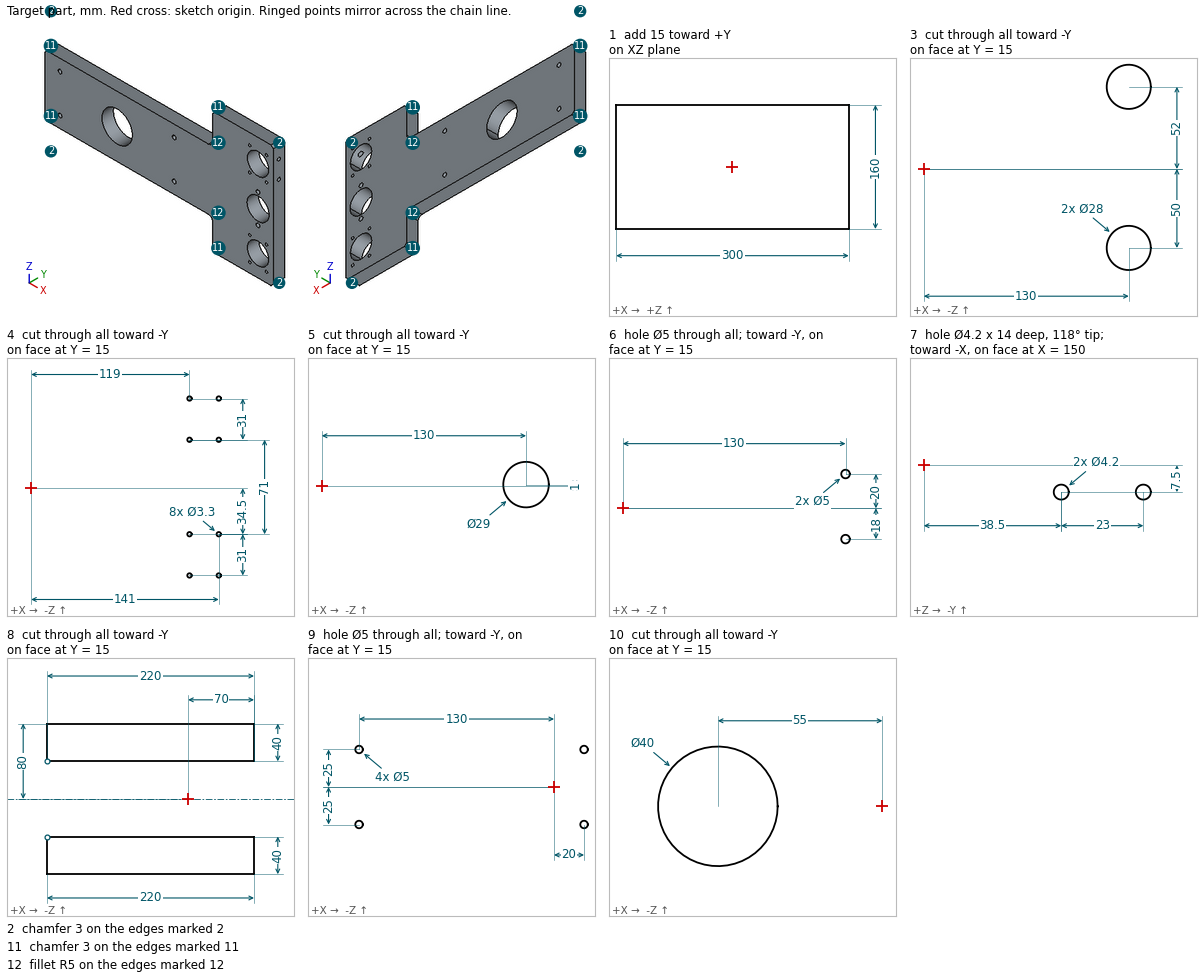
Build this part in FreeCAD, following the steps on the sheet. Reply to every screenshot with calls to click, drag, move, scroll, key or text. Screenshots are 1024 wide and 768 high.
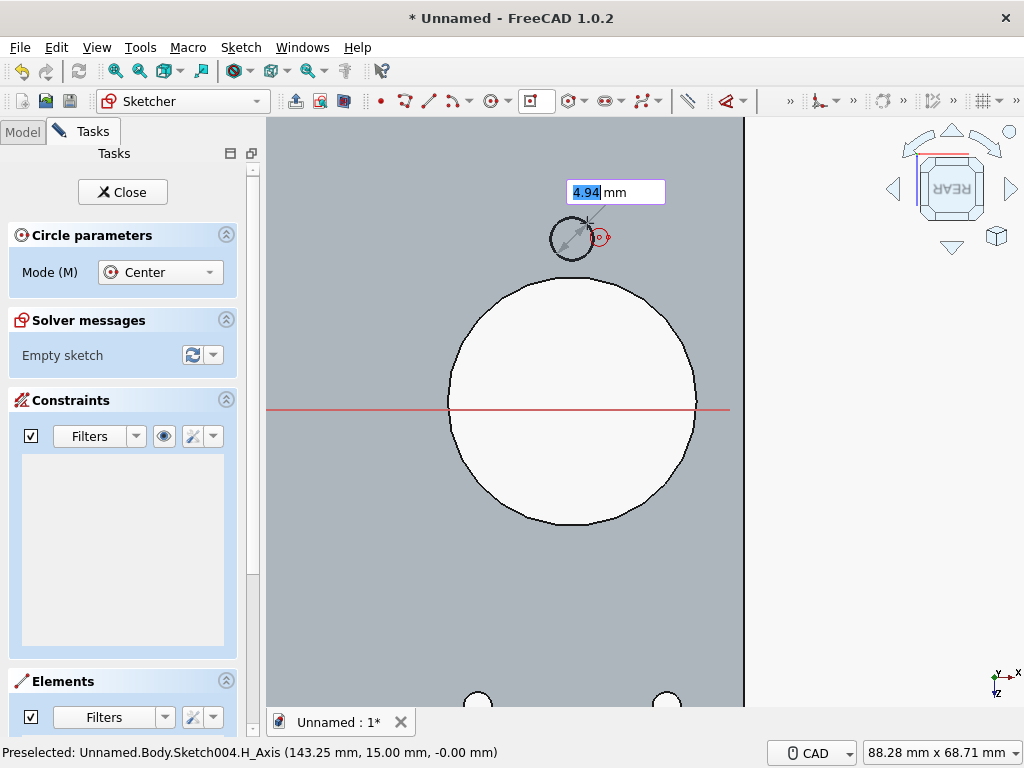
text(5)
key(Return)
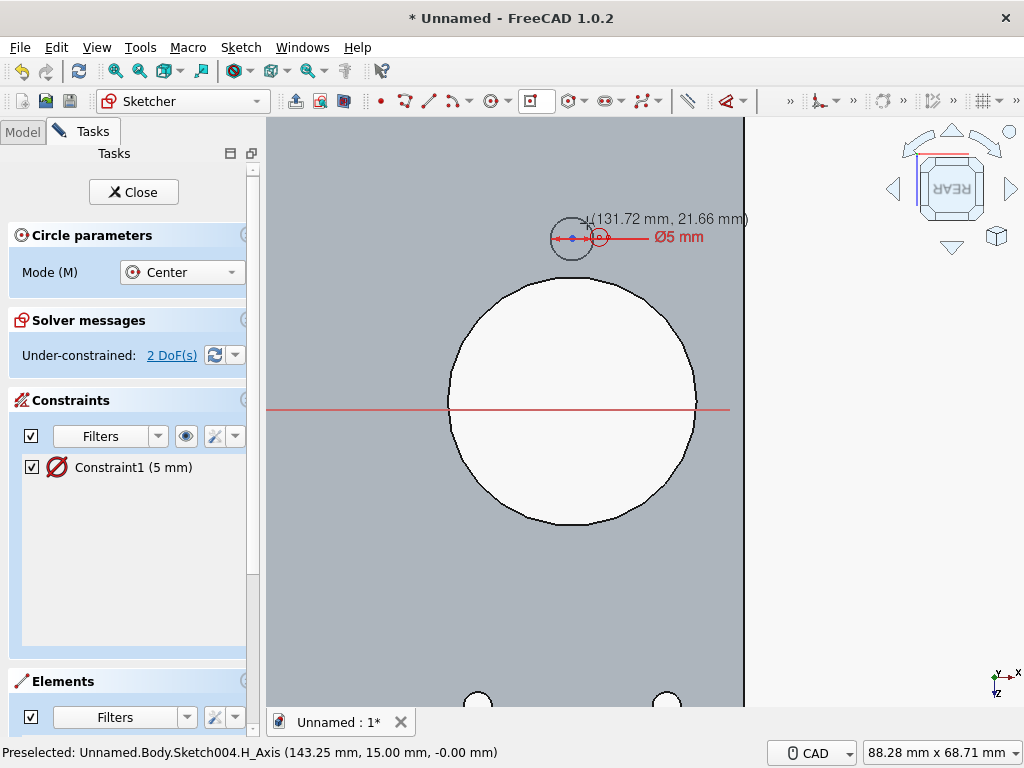
click(572, 565)
move(587, 549)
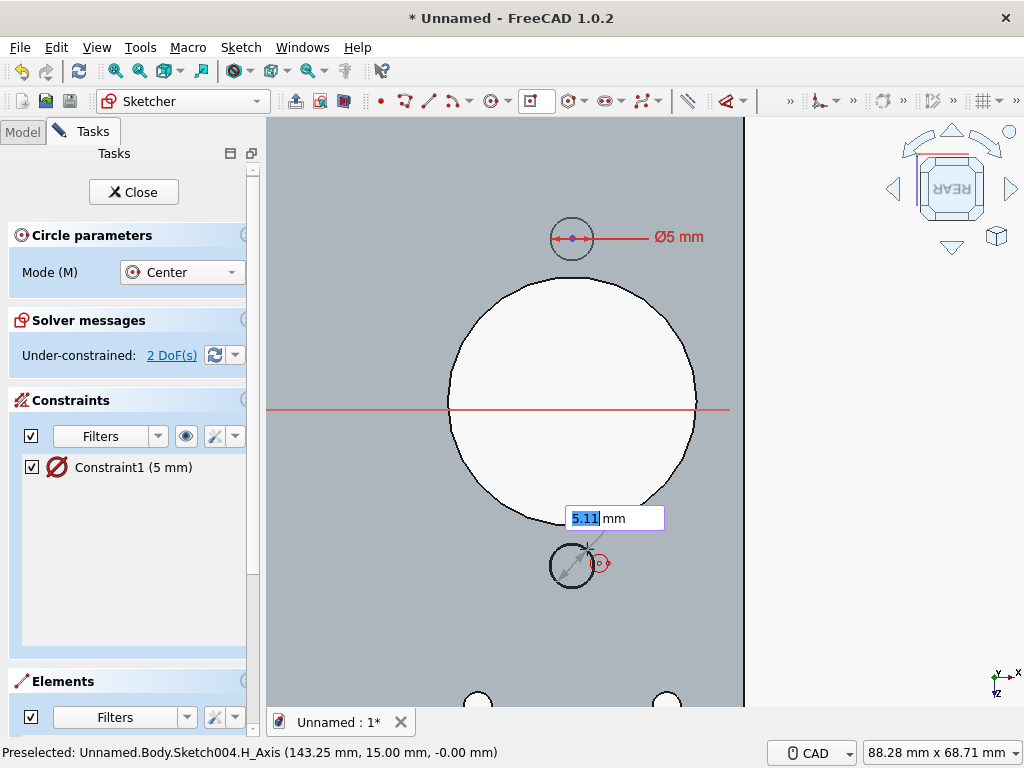
text(5)
key(Return)
key(Escape)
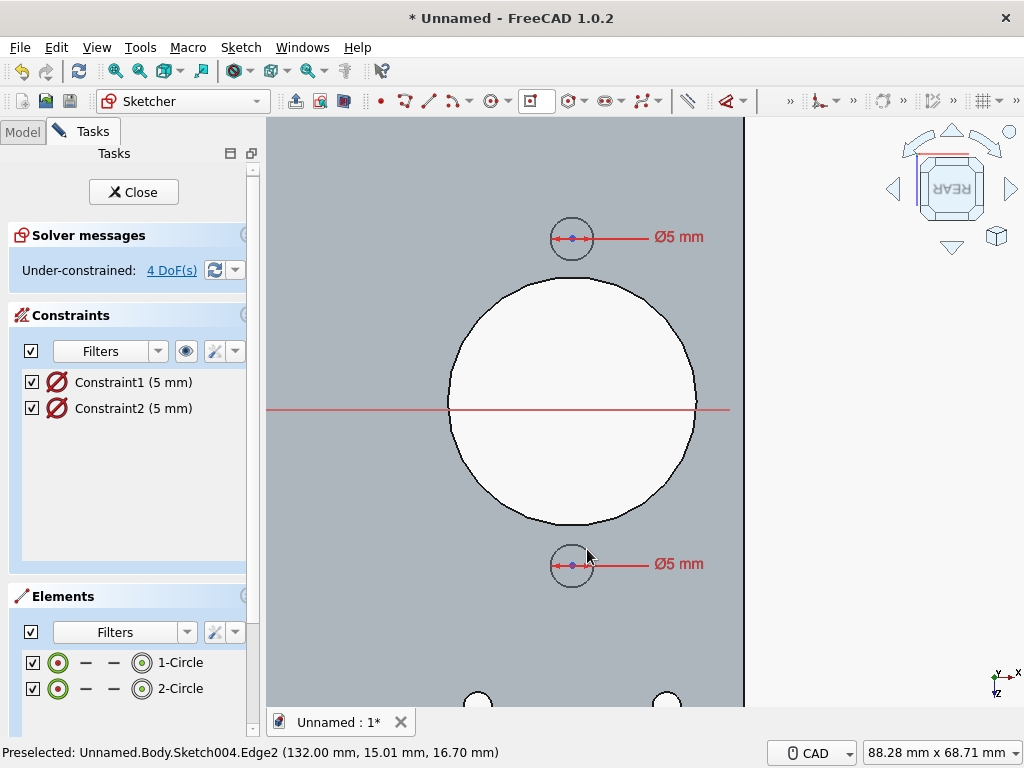
click(572, 239)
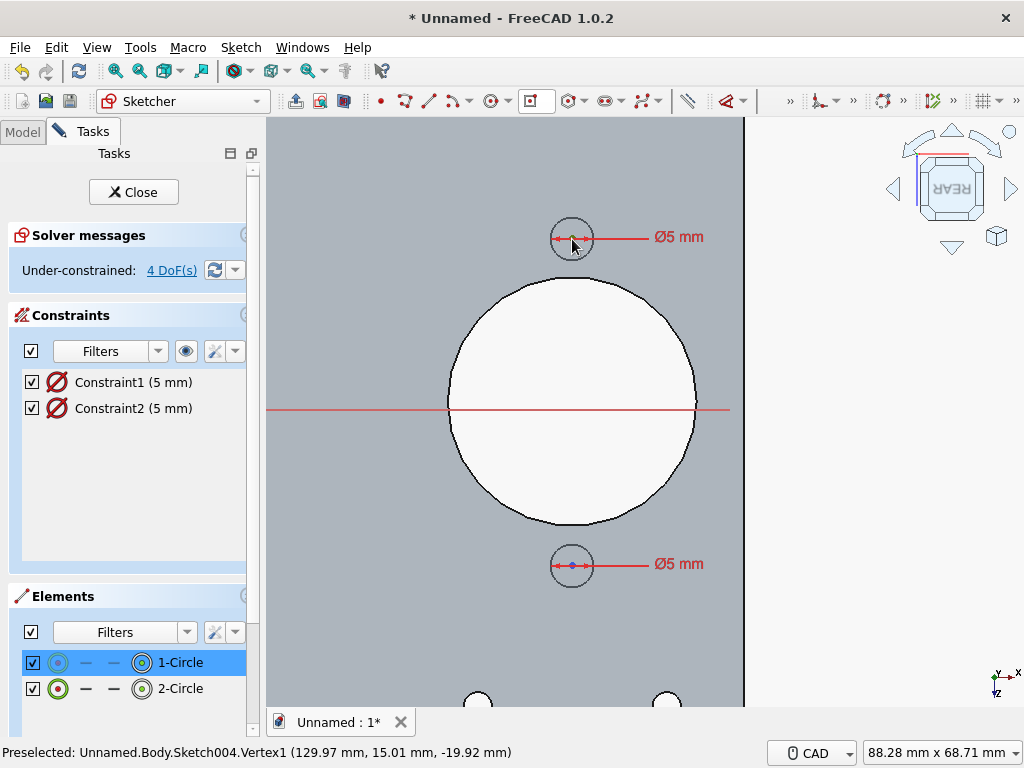
click(572, 566)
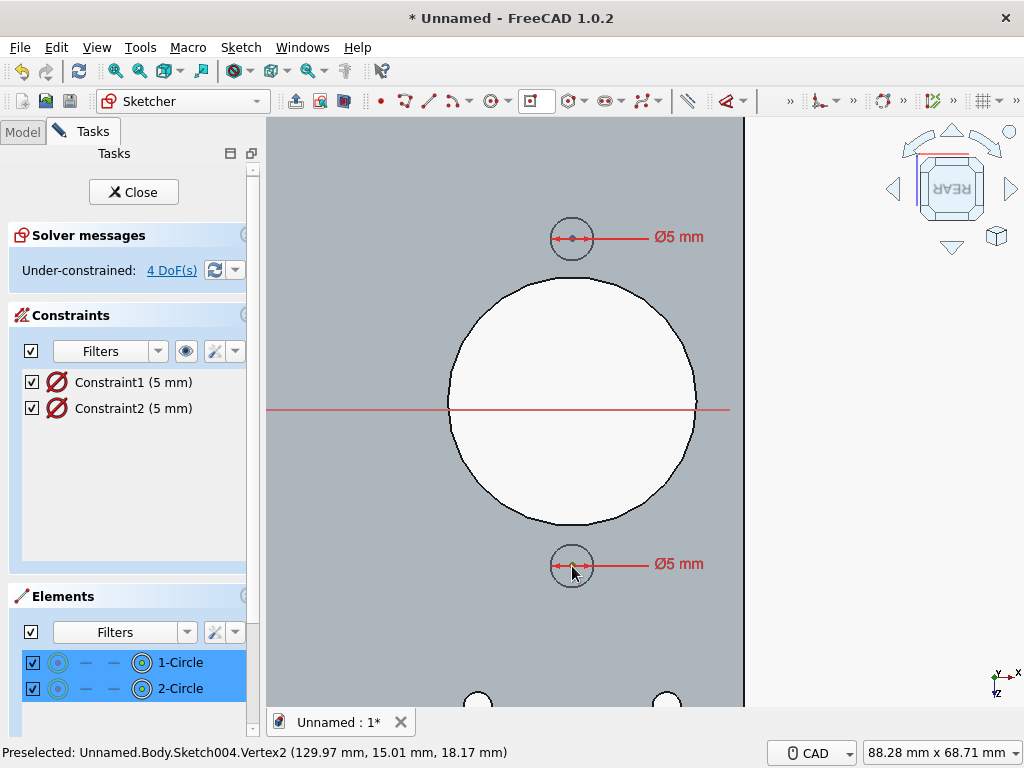
key(v)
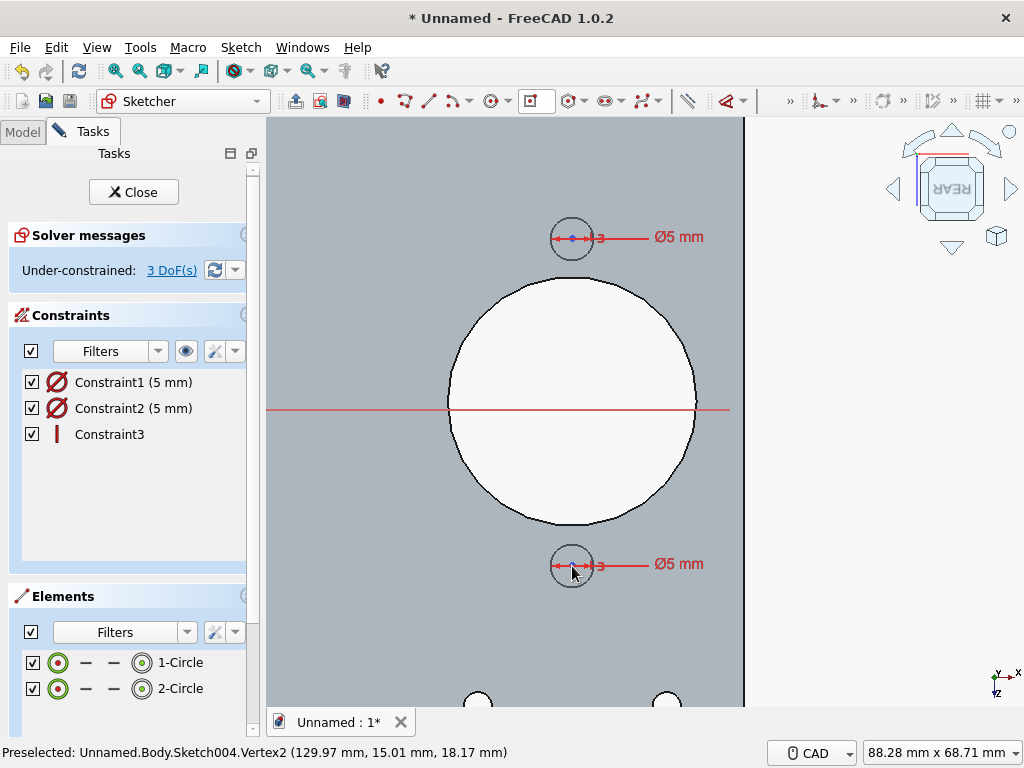
click(726, 102)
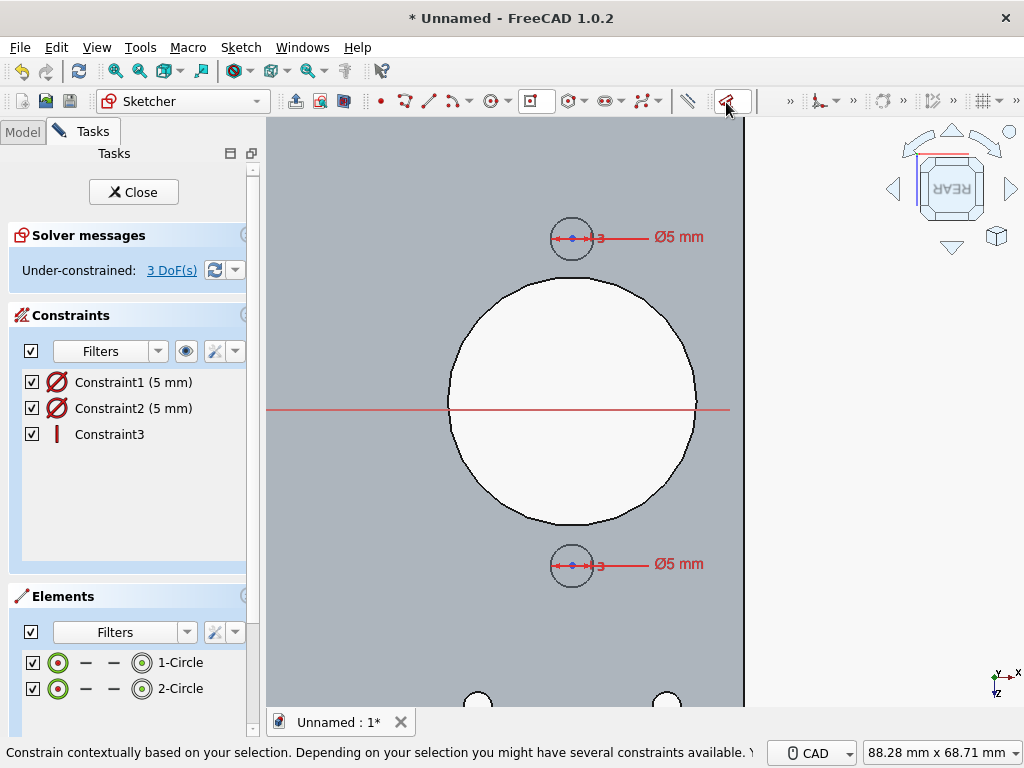
click(572, 239)
click(606, 325)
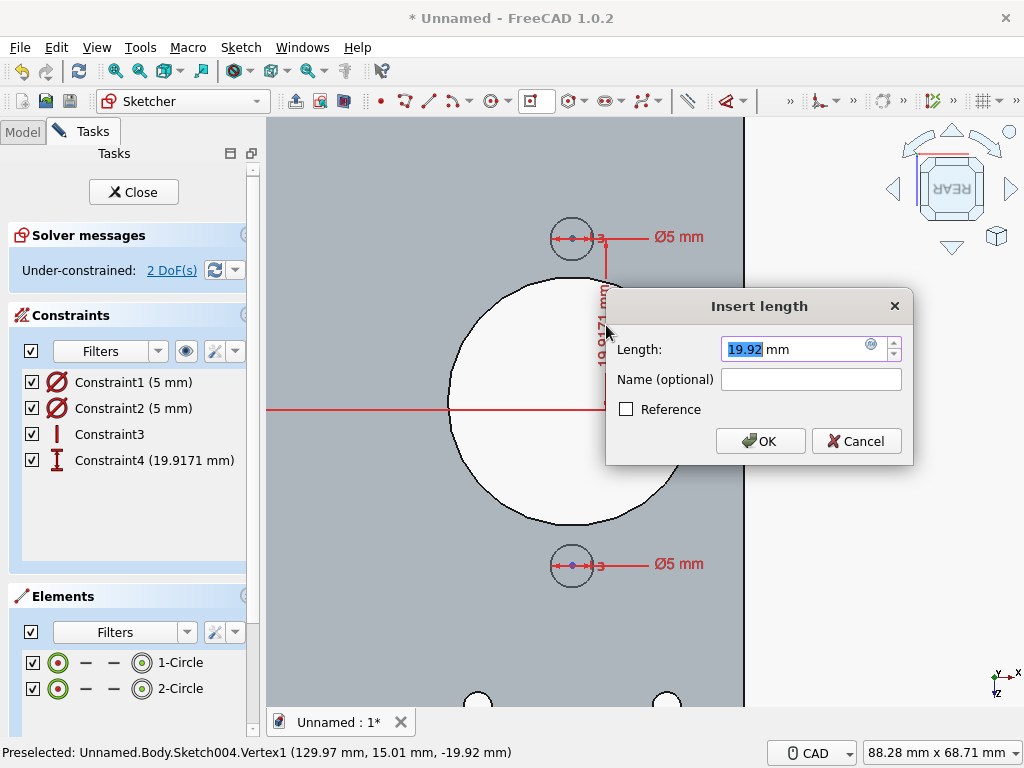
text(20)
key(Return)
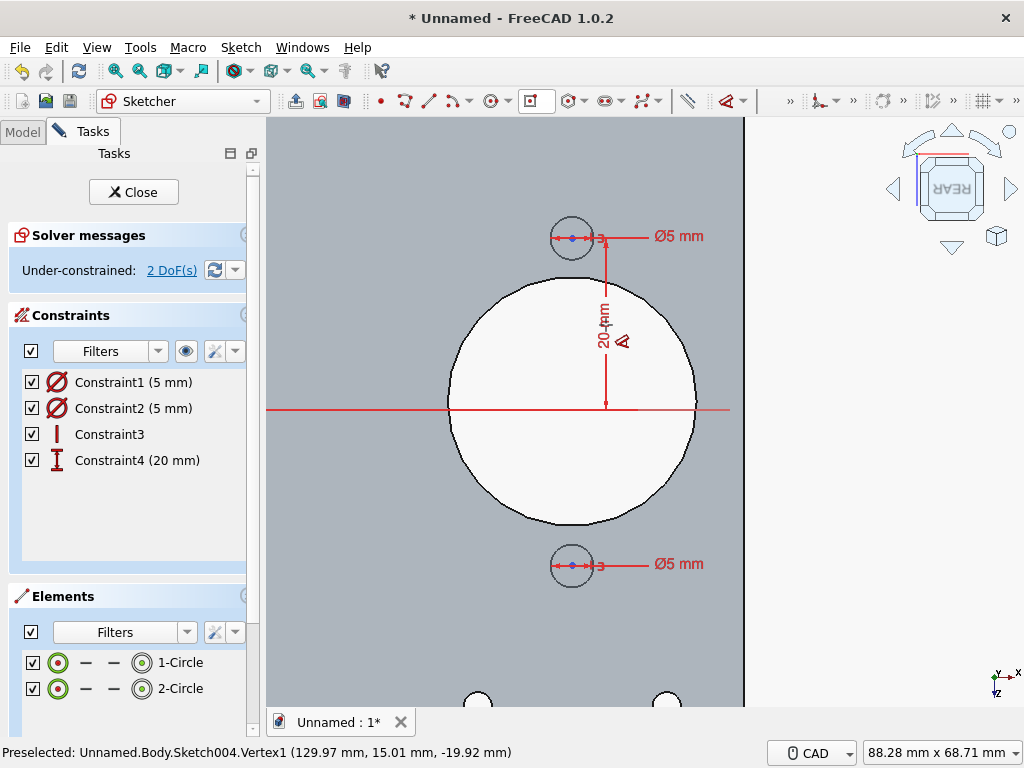
click(572, 566)
click(606, 488)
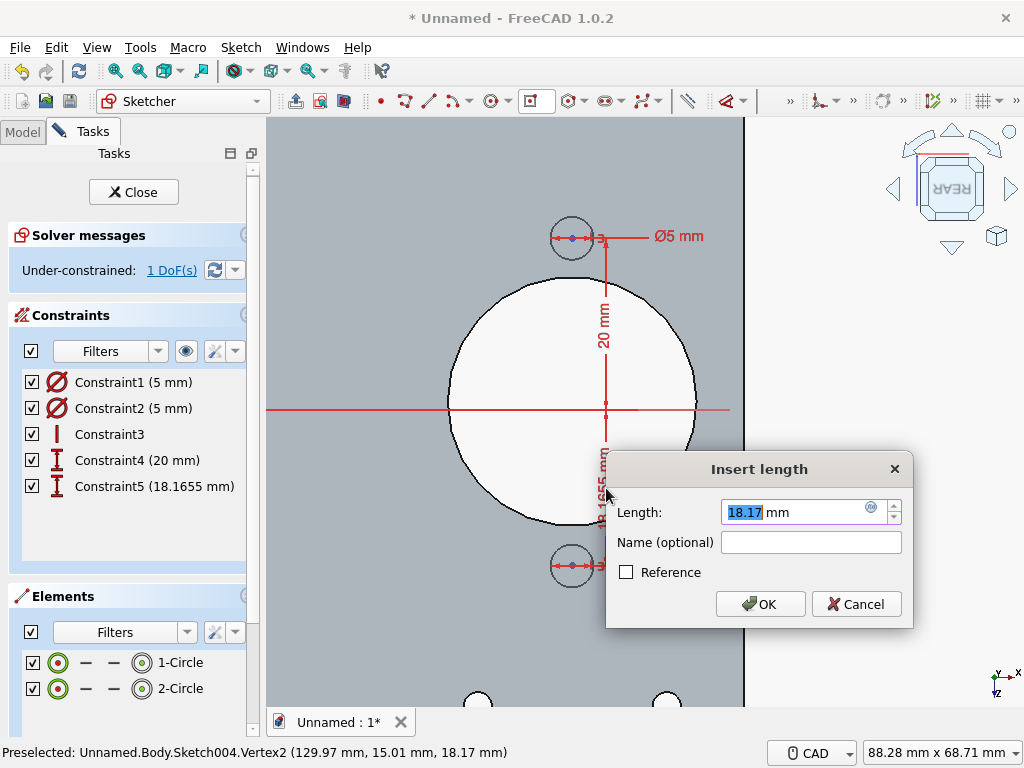
text(18)
key(Return)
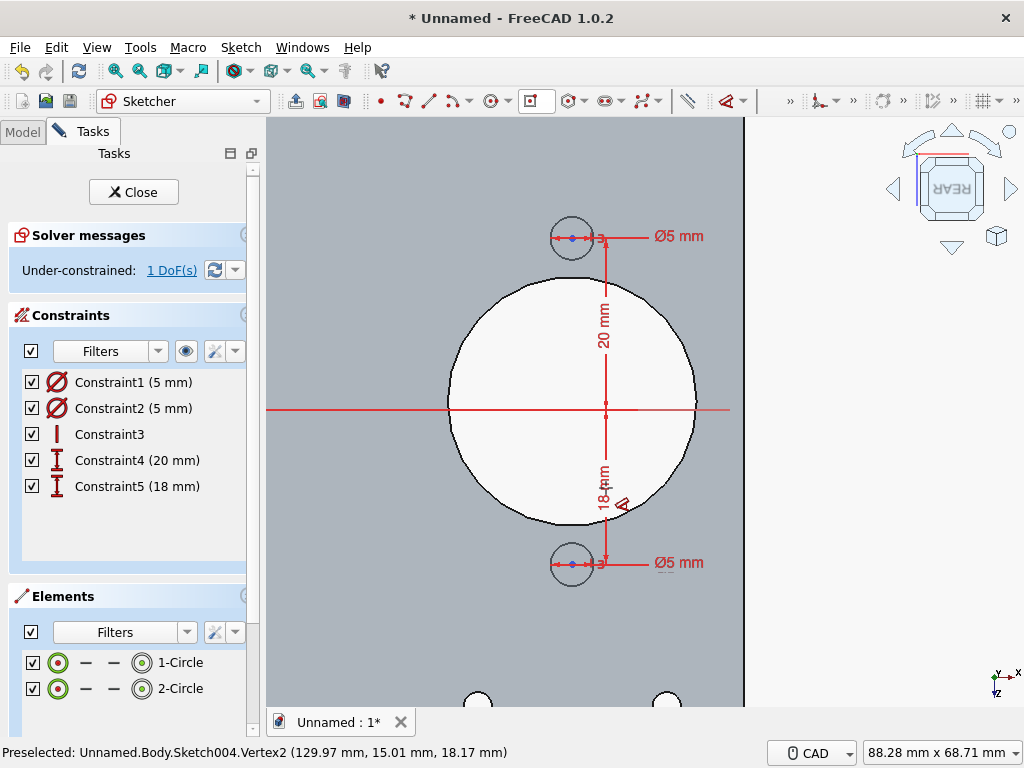
click(572, 238)
click(433, 204)